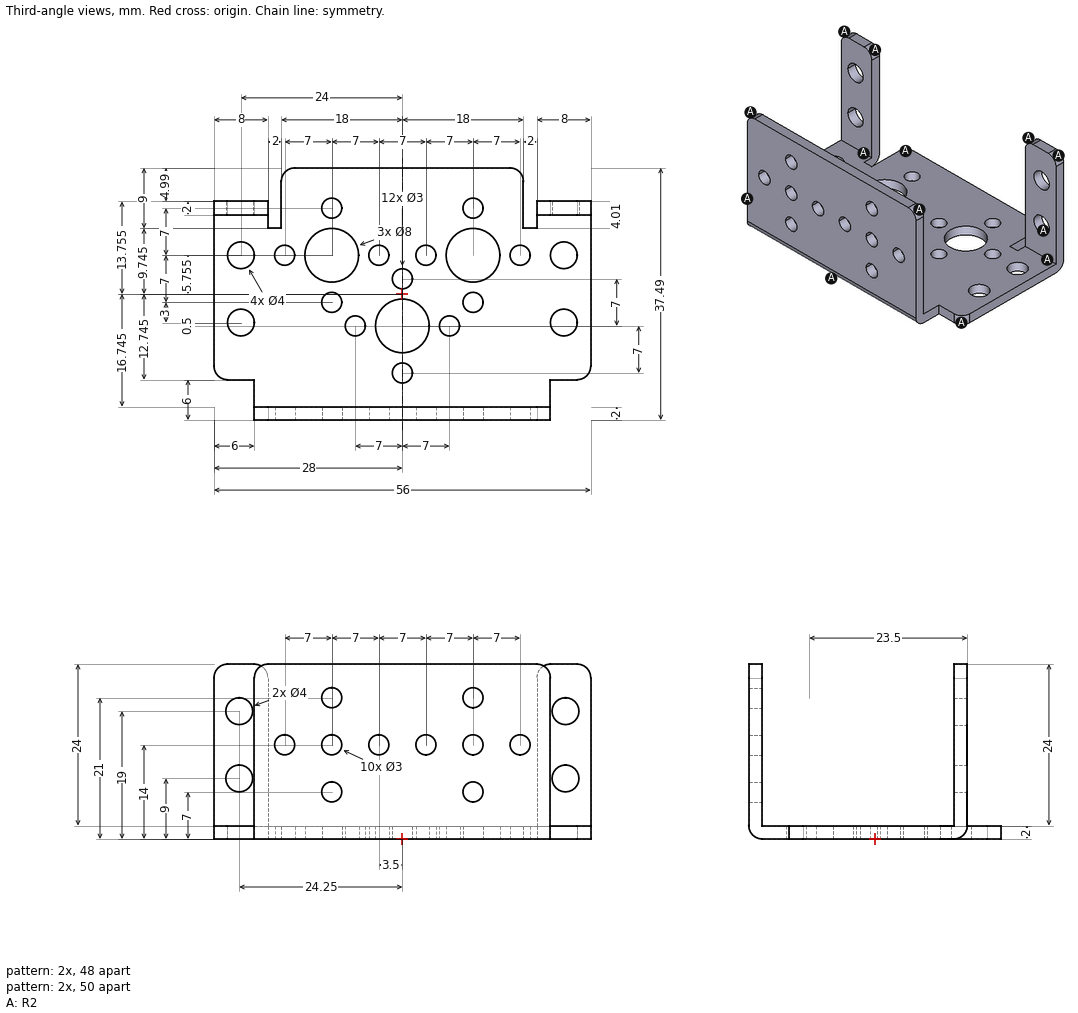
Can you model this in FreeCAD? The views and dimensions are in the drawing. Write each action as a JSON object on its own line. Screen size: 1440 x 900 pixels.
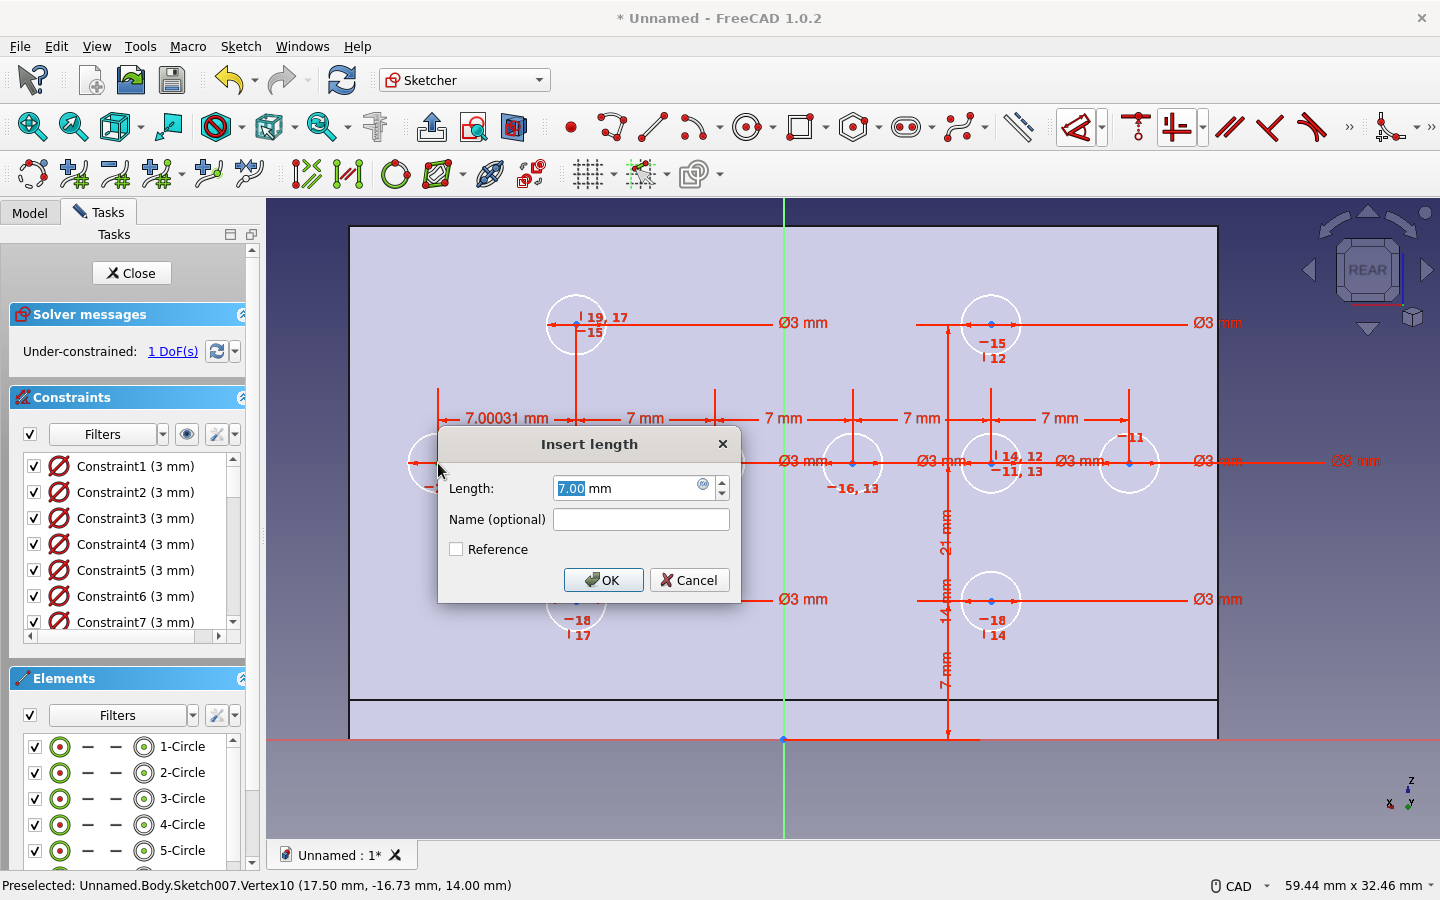
{"action": "type", "text": "7"}
{"action": "key", "text": "Return"}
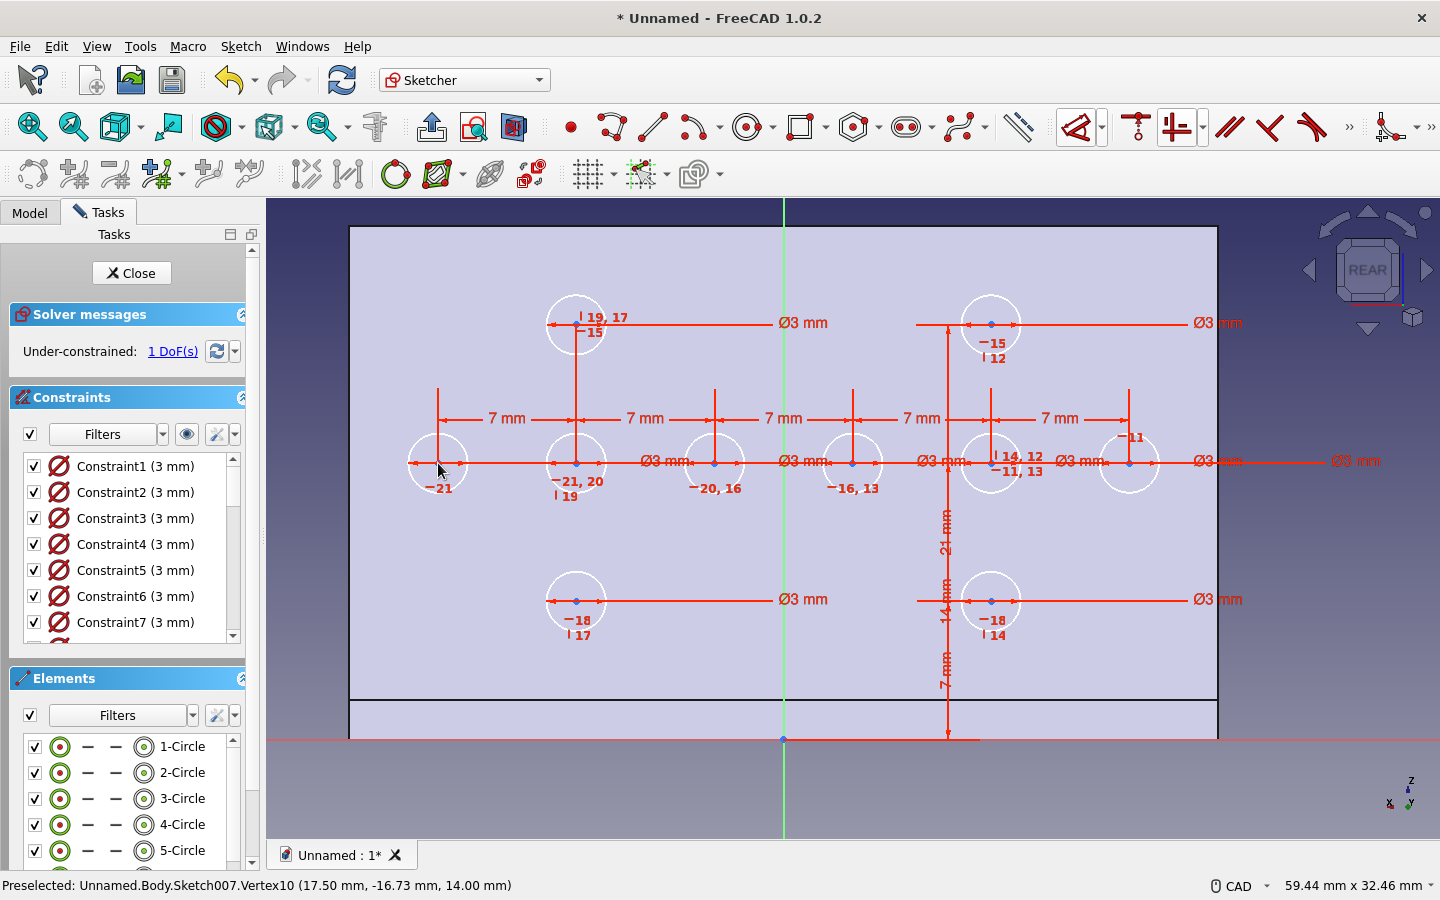
{"action": "left_click", "coordinate": [853, 463]}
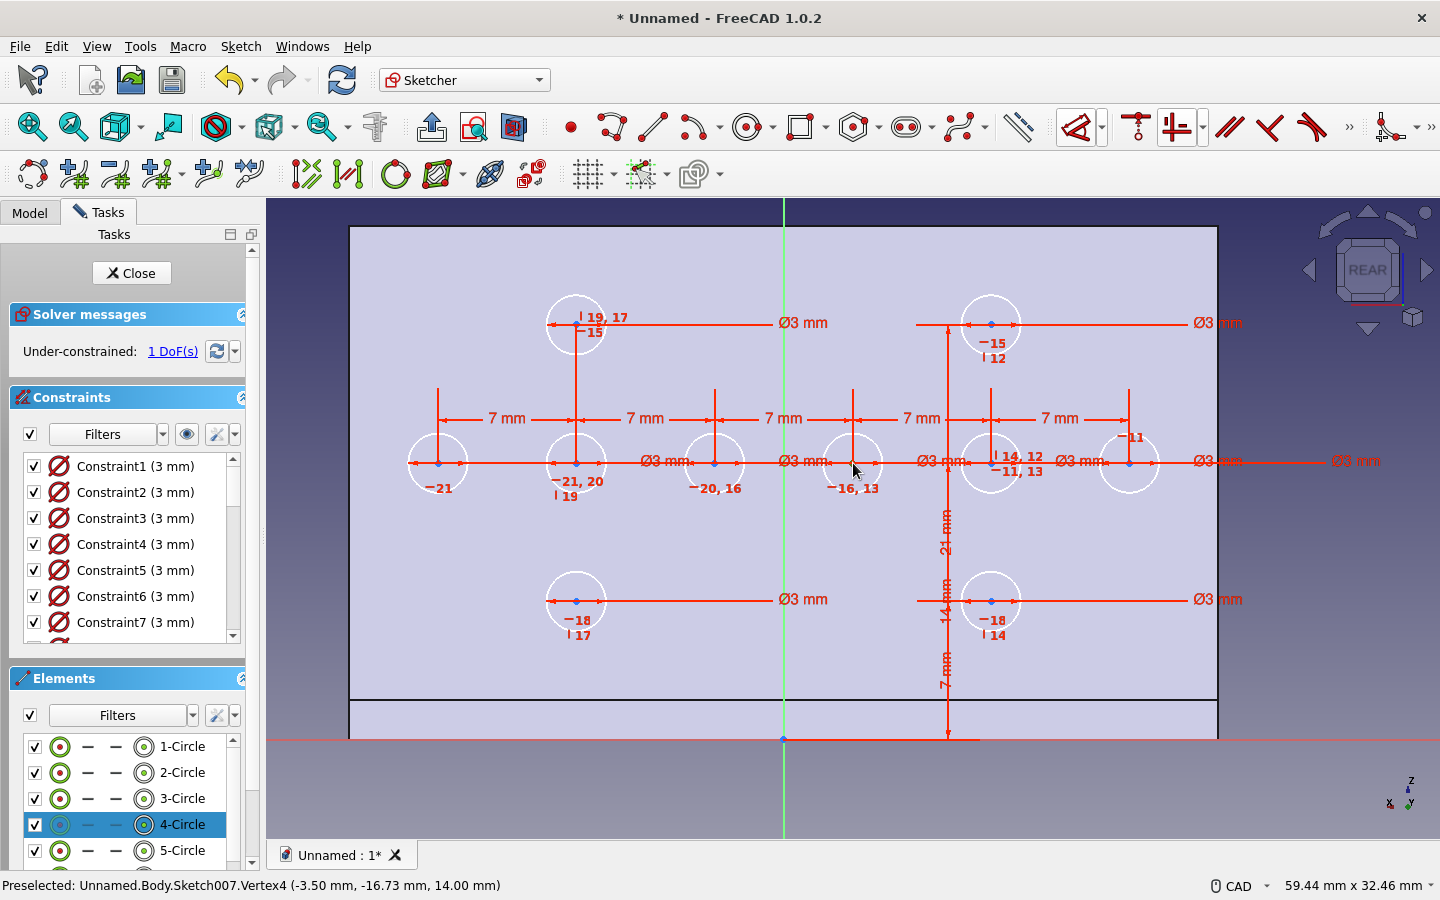
{"action": "key", "text": "l"}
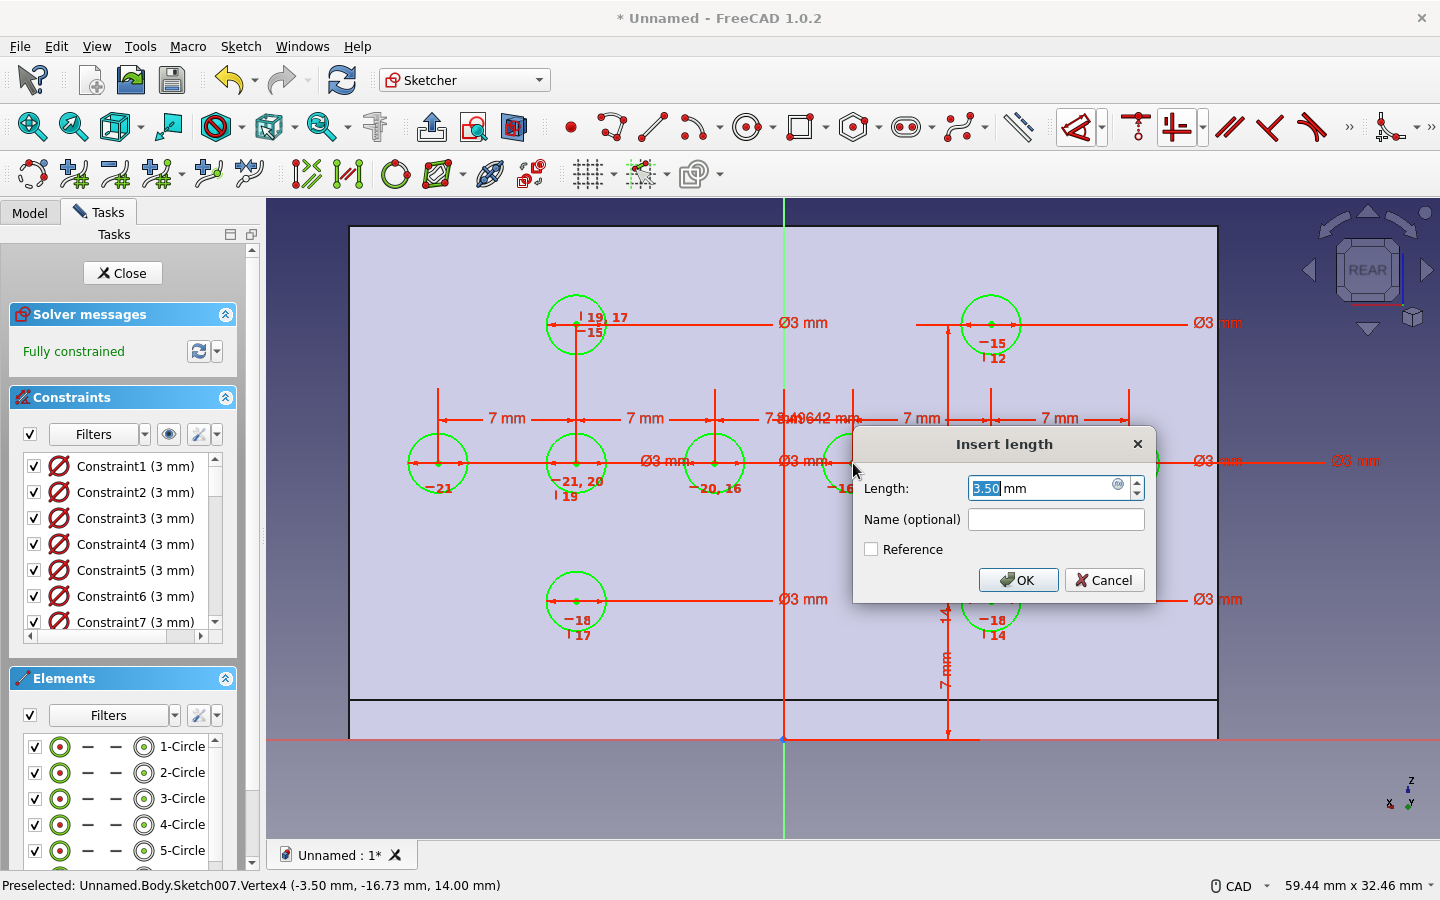
{"action": "type", "text": "3.5"}
{"action": "key", "text": "Return"}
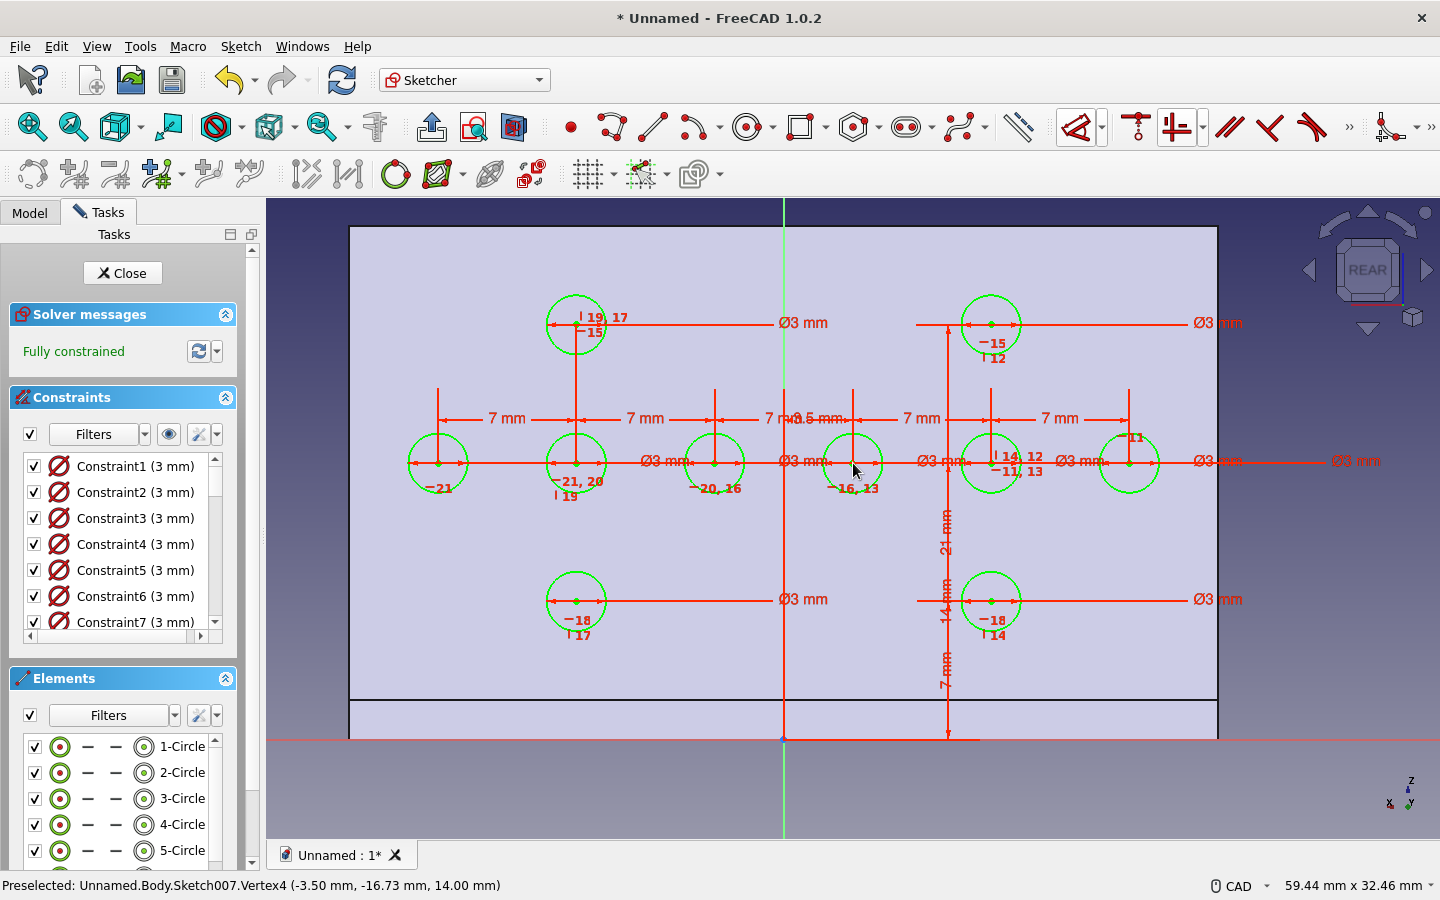
{"action": "left_click", "coordinate": [123, 273]}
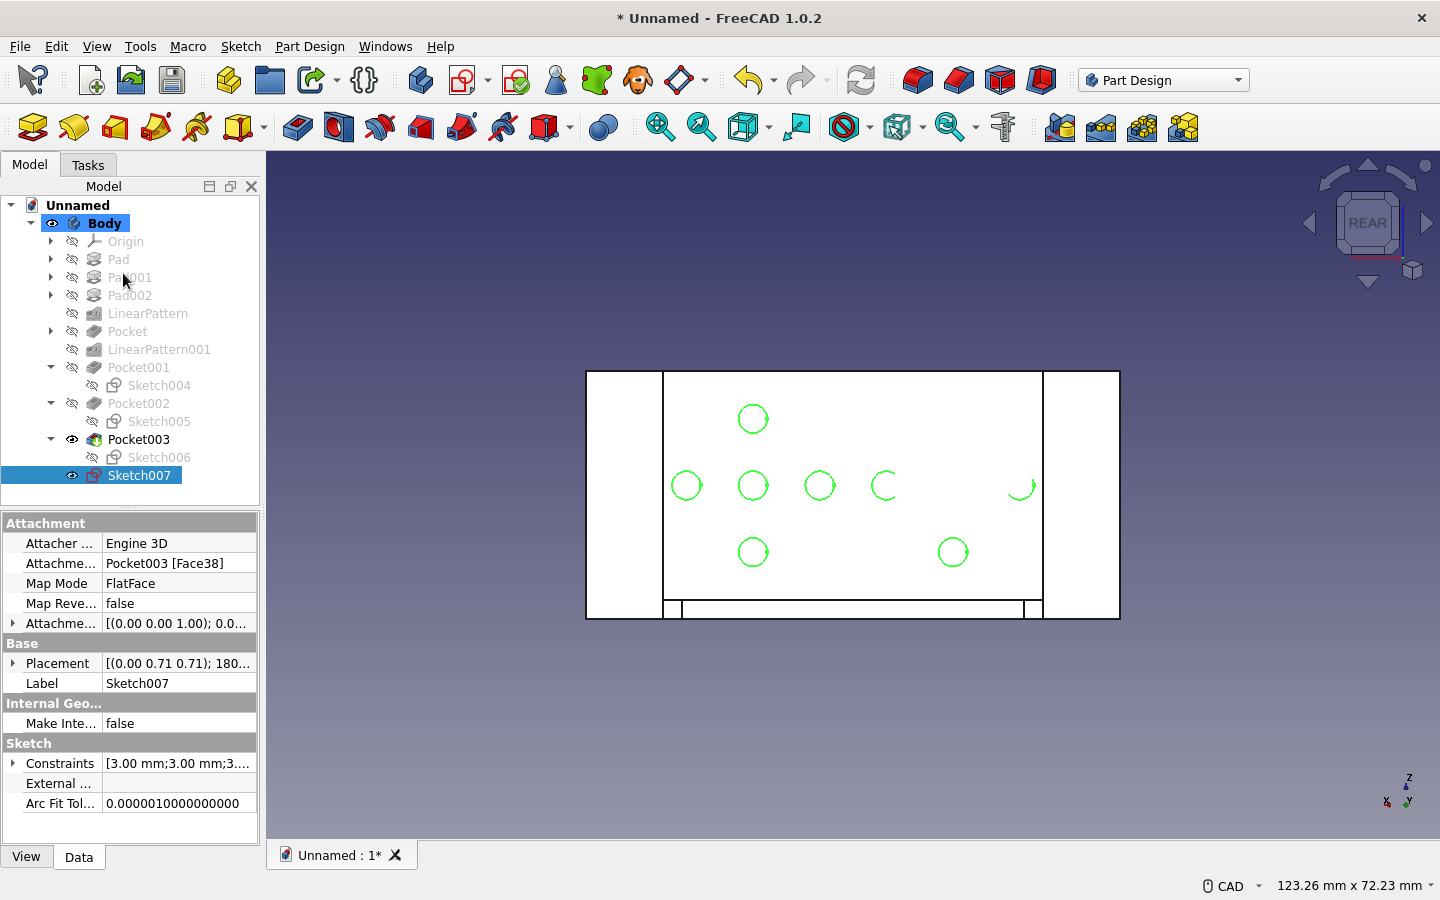
{"action": "left_click", "coordinate": [298, 128]}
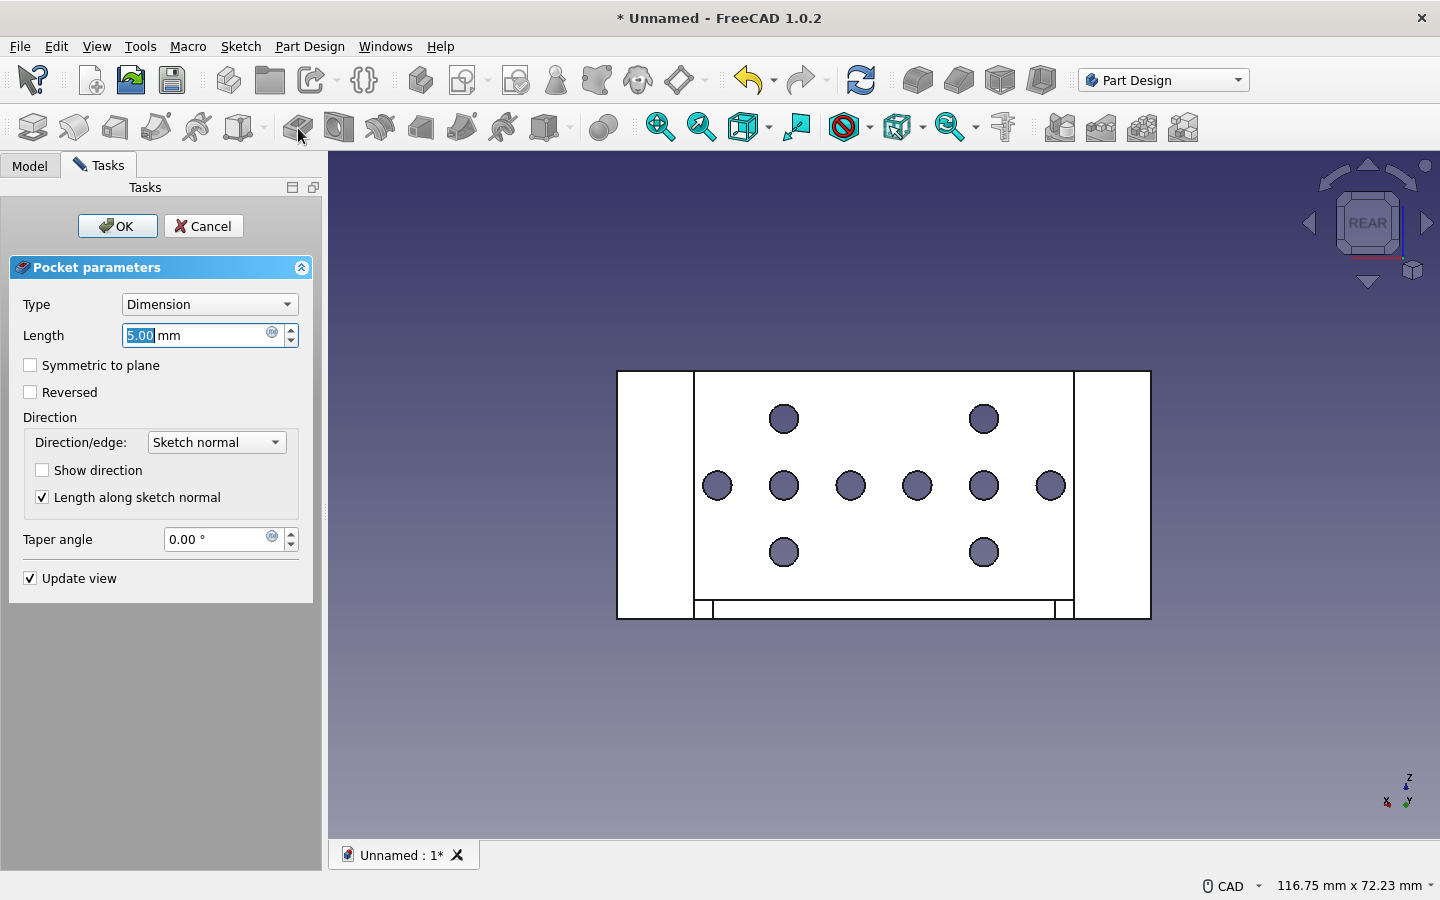
{"action": "left_click", "coordinate": [210, 304]}